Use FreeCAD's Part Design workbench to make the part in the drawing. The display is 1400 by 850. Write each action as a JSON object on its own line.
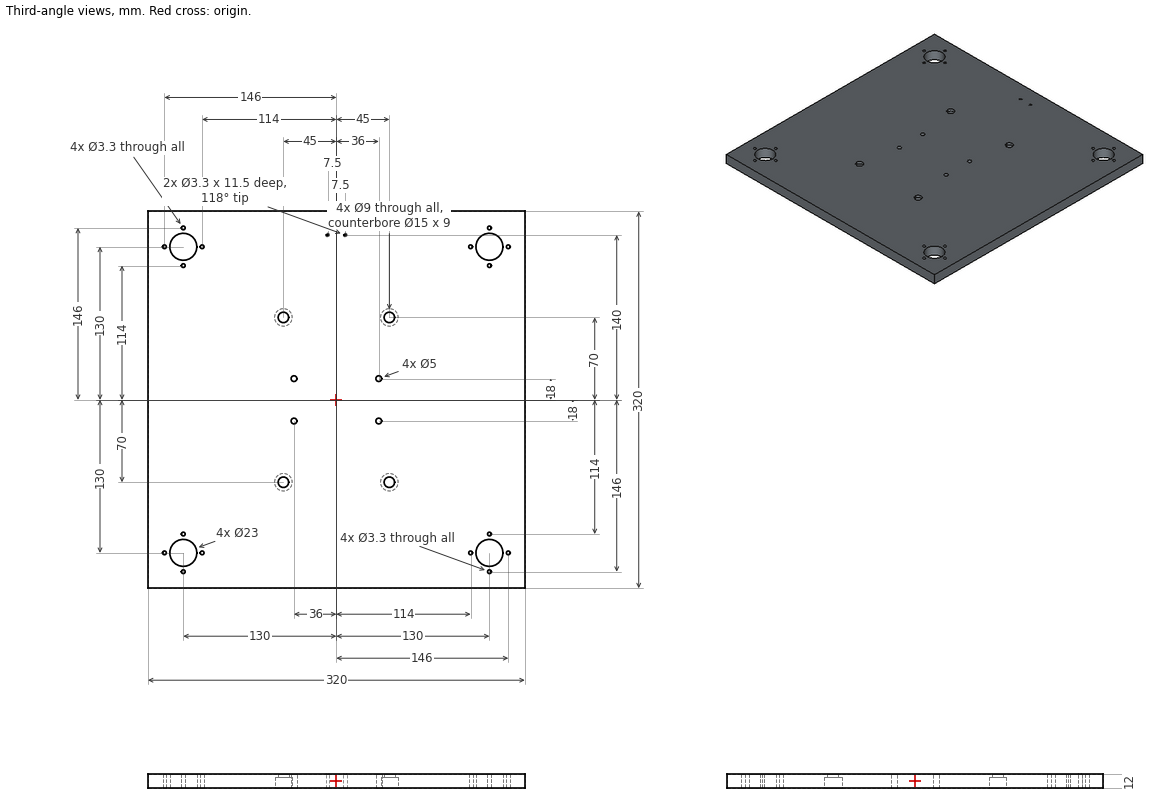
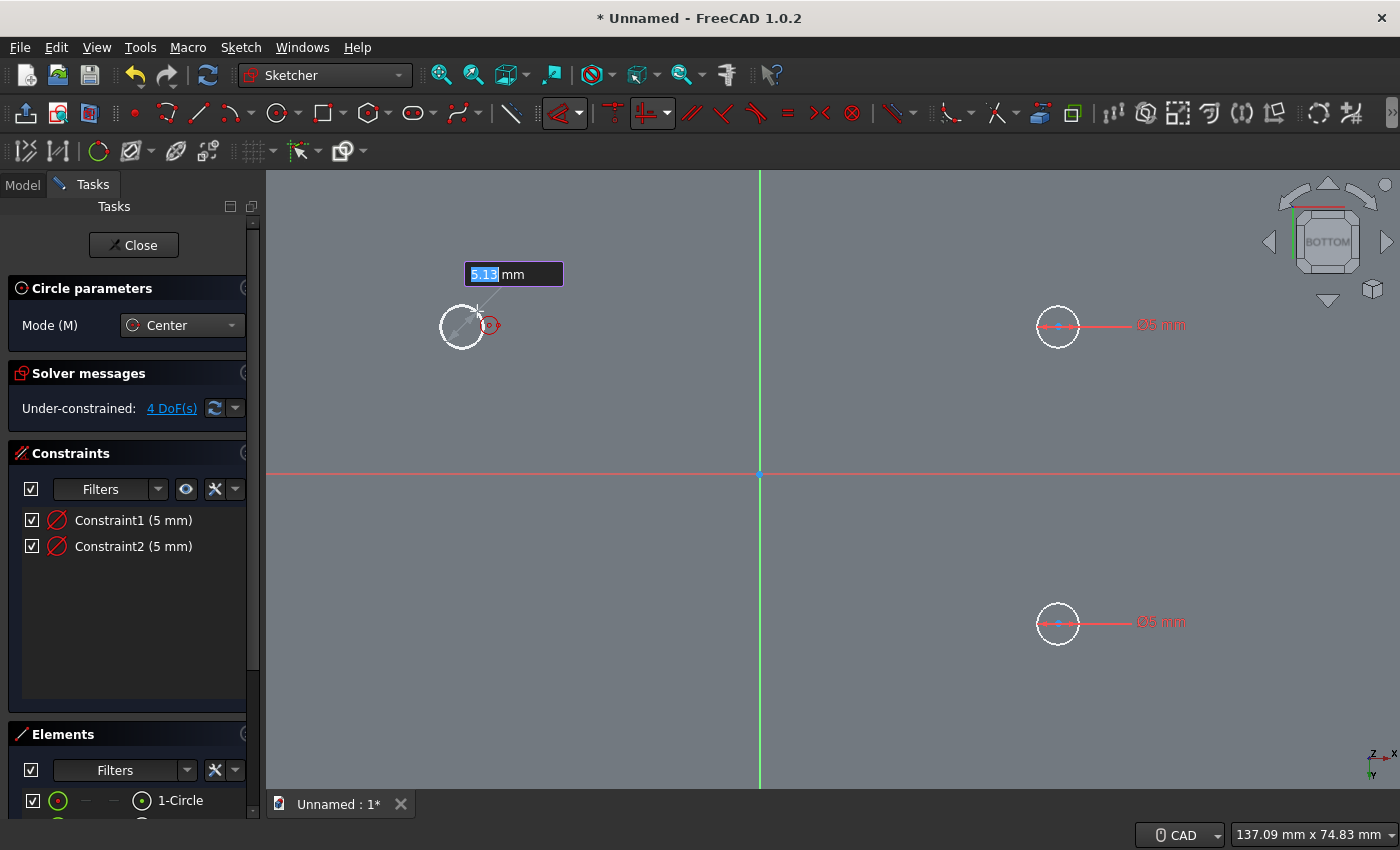
{"action": "type", "text": "5"}
{"action": "key", "text": "Return"}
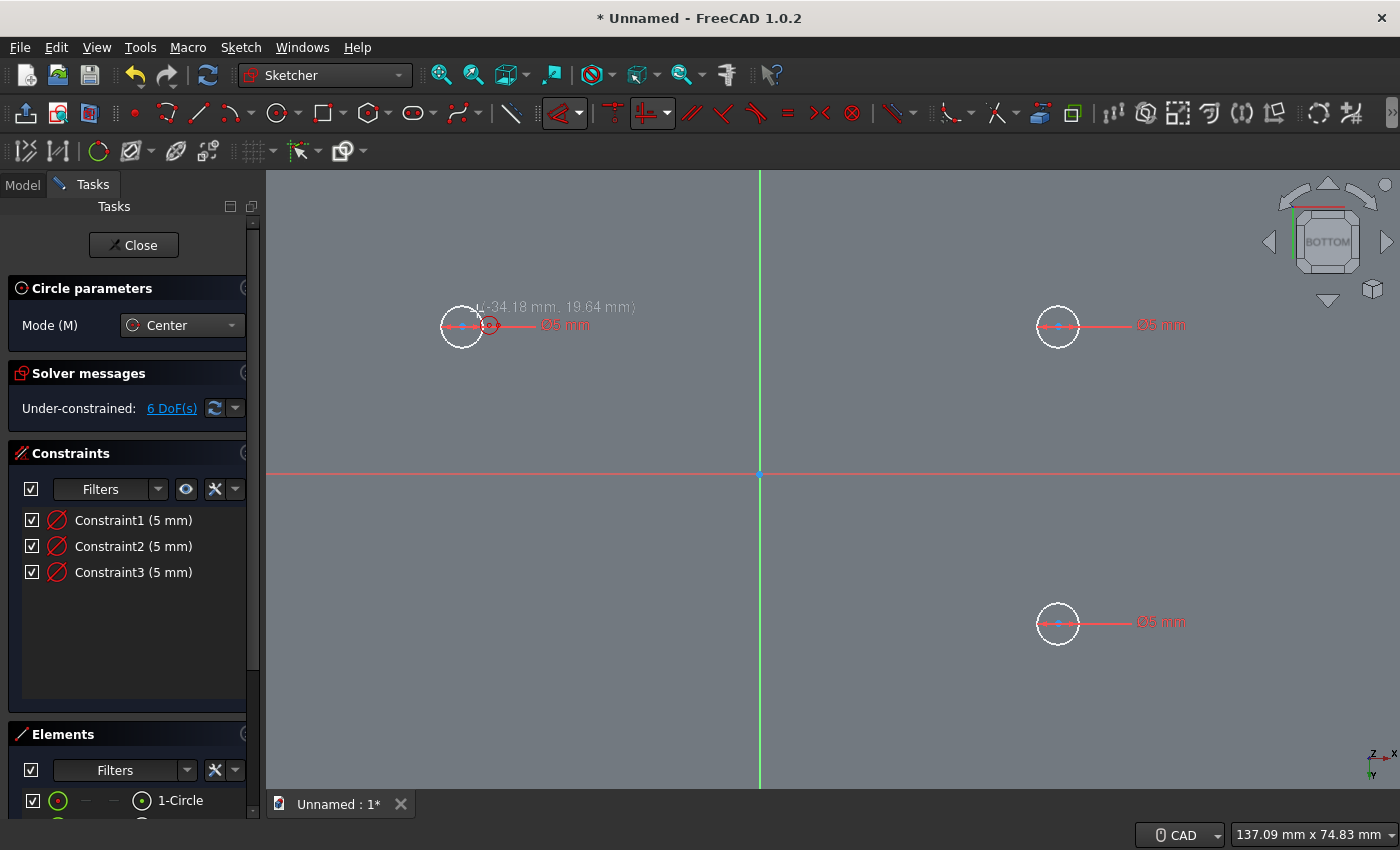
{"action": "left_click", "coordinate": [462, 623]}
{"action": "mouse_move", "coordinate": [477, 609]}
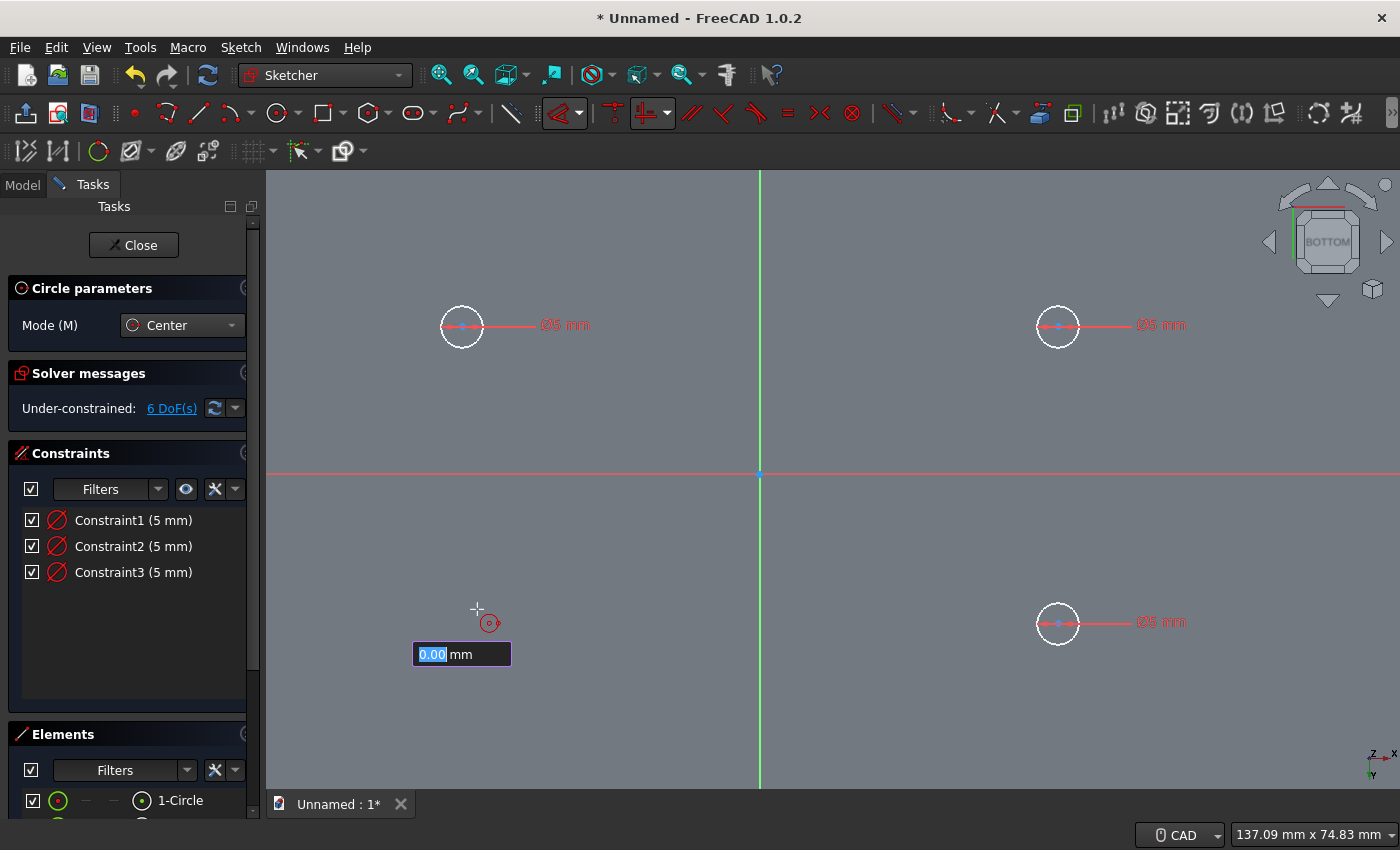
{"action": "type", "text": "5"}
{"action": "key", "text": "Return"}
{"action": "key", "text": "Escape"}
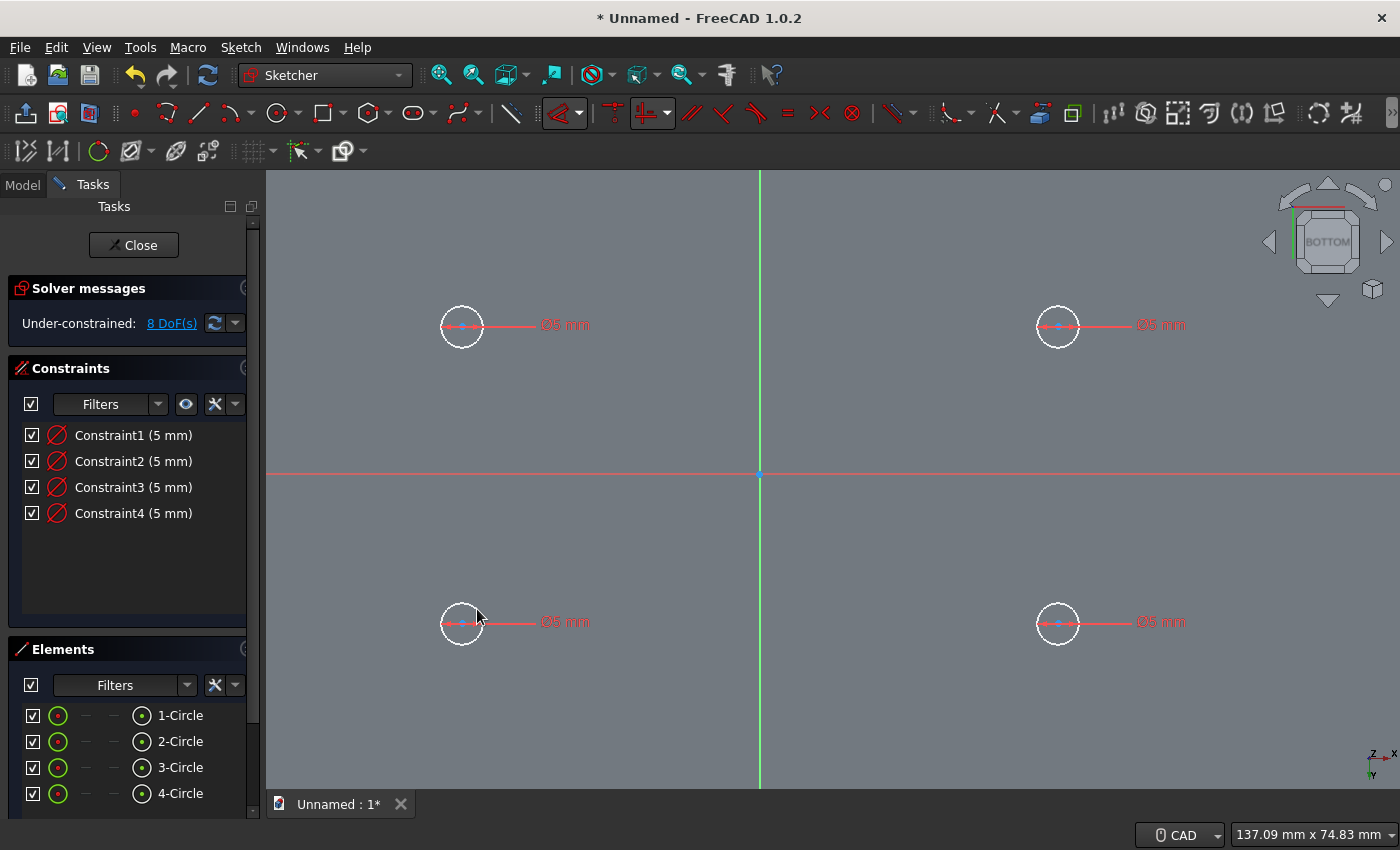
{"action": "left_click", "coordinate": [1058, 624]}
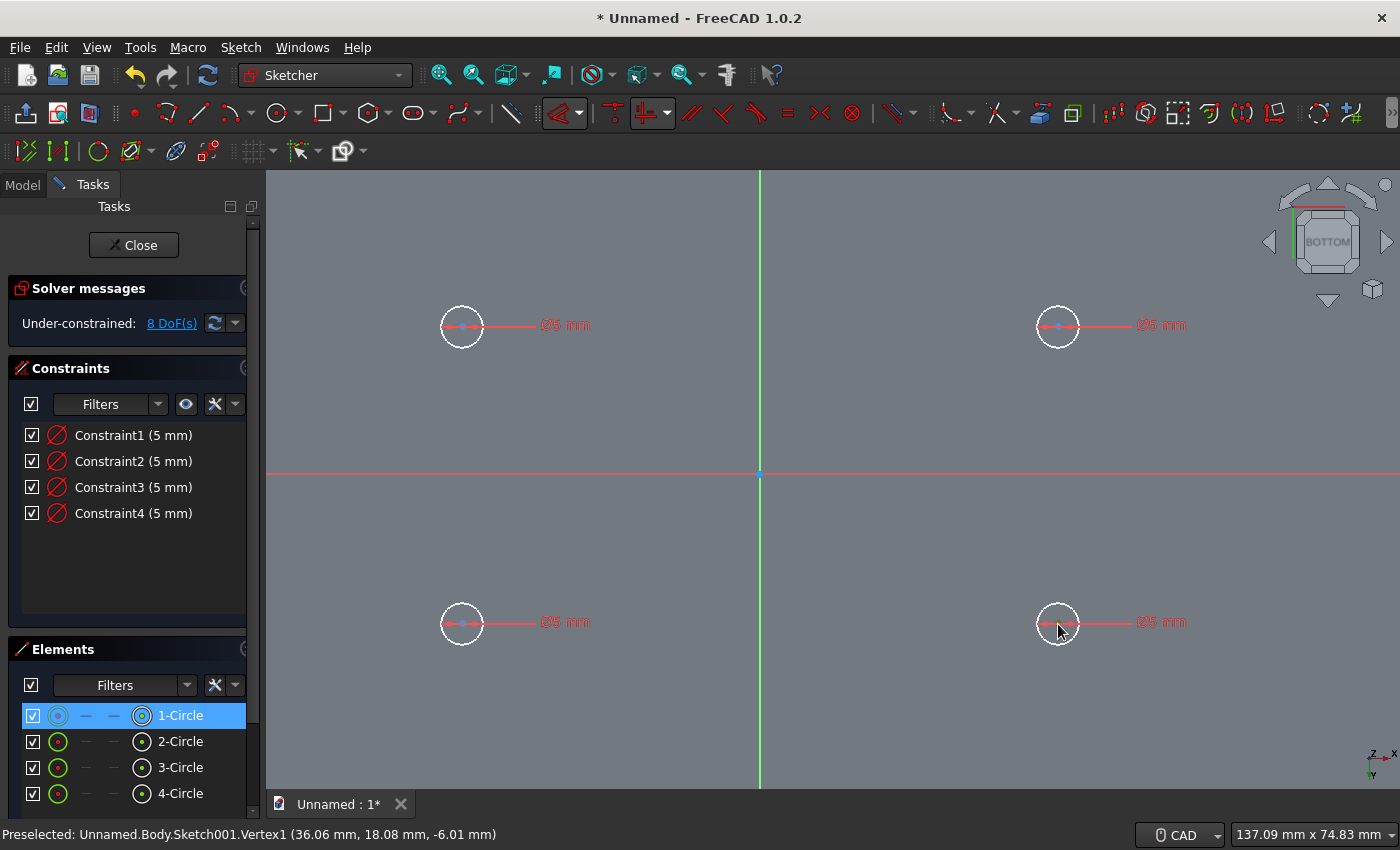
{"action": "left_click", "coordinate": [1058, 327]}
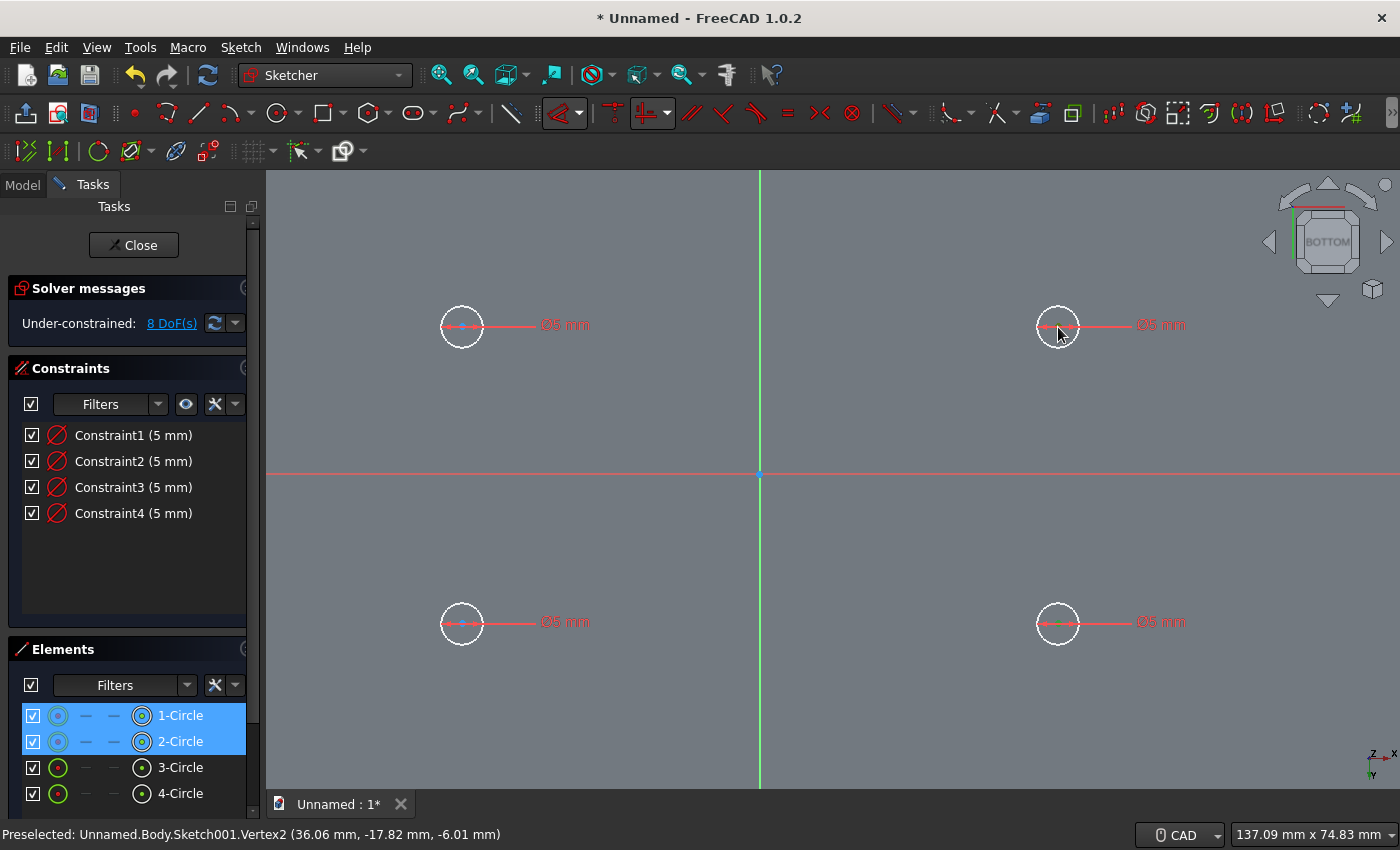
{"action": "left_click", "coordinate": [670, 114]}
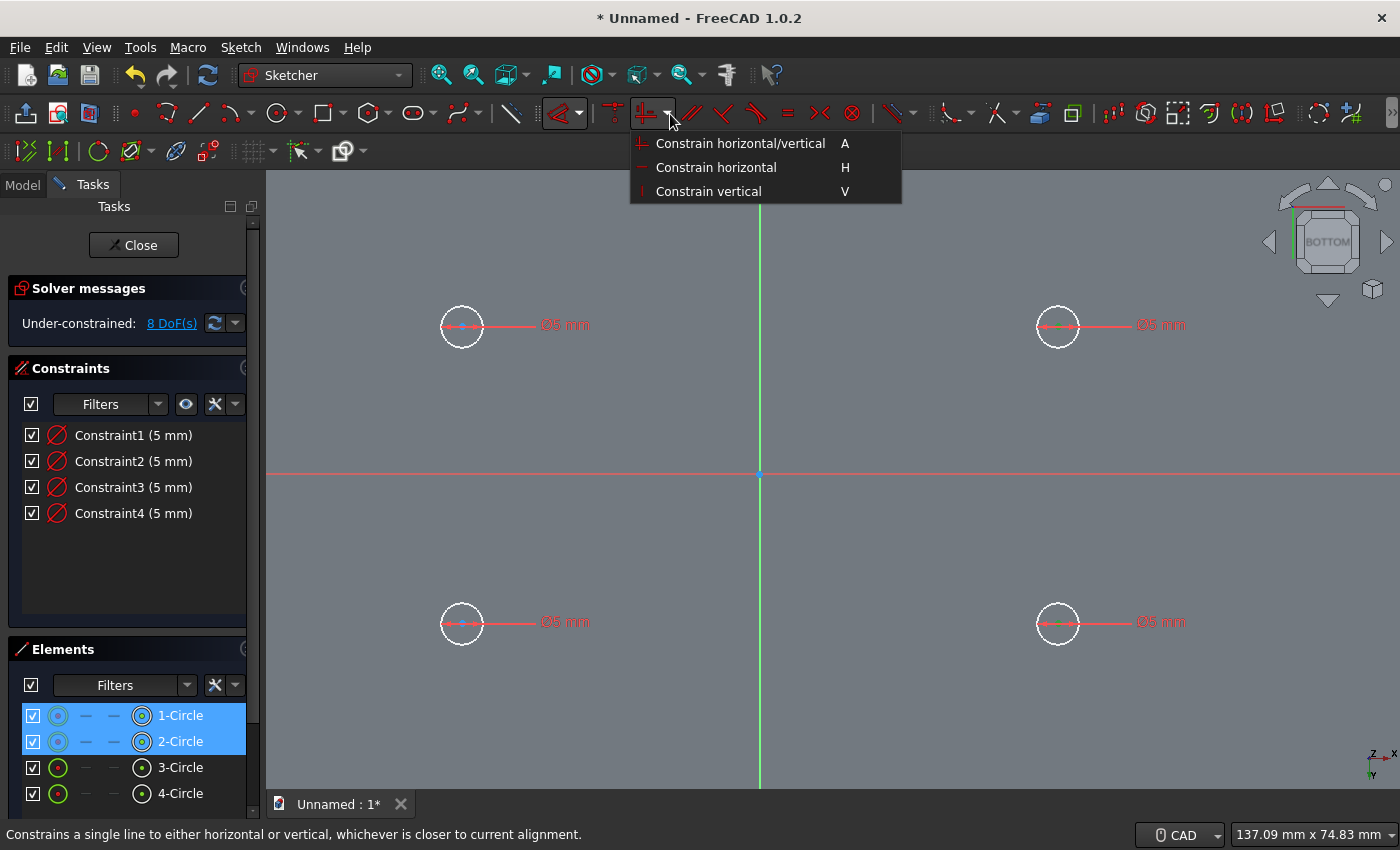
{"action": "left_click", "coordinate": [766, 191]}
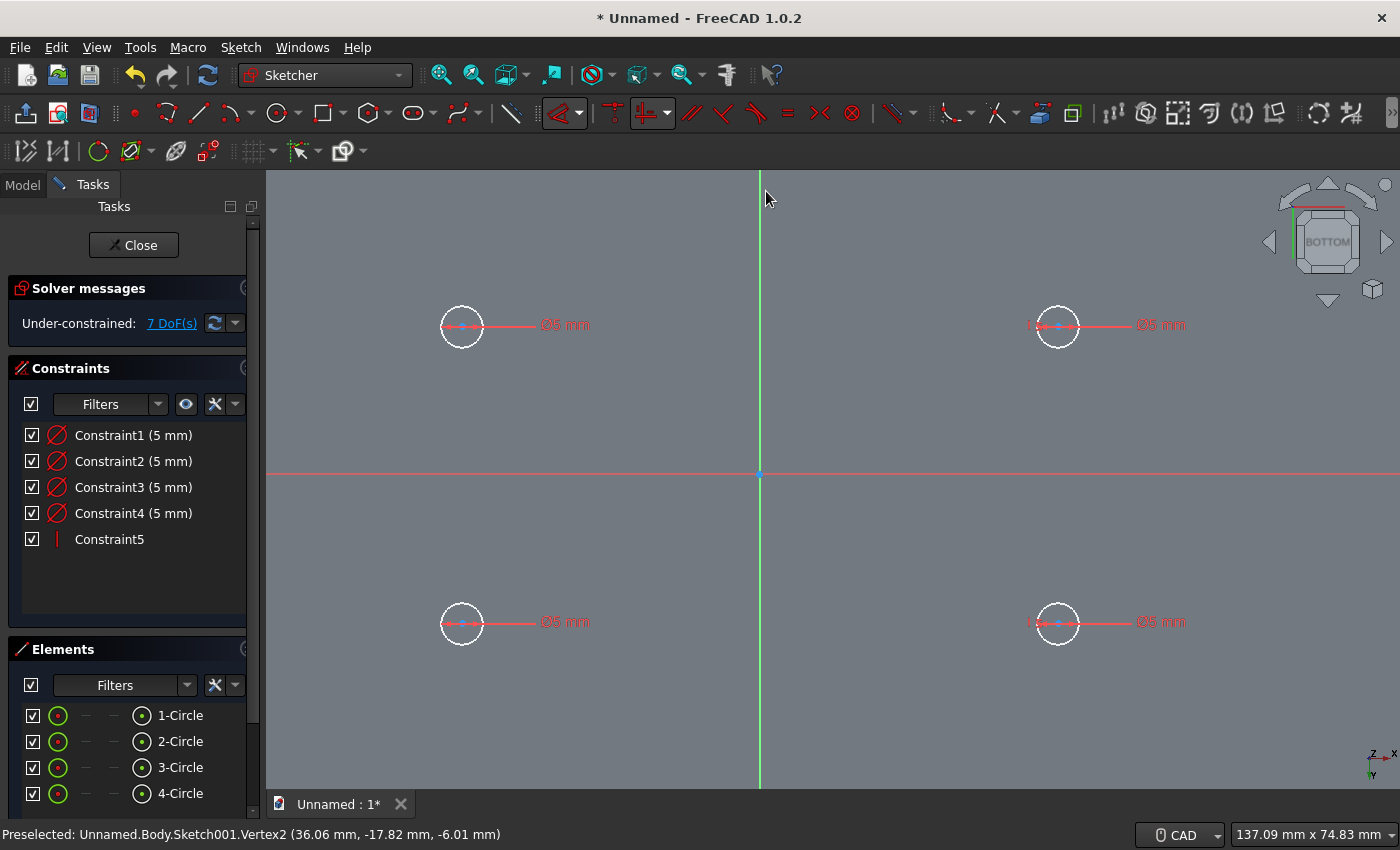
{"action": "left_click", "coordinate": [1058, 327]}